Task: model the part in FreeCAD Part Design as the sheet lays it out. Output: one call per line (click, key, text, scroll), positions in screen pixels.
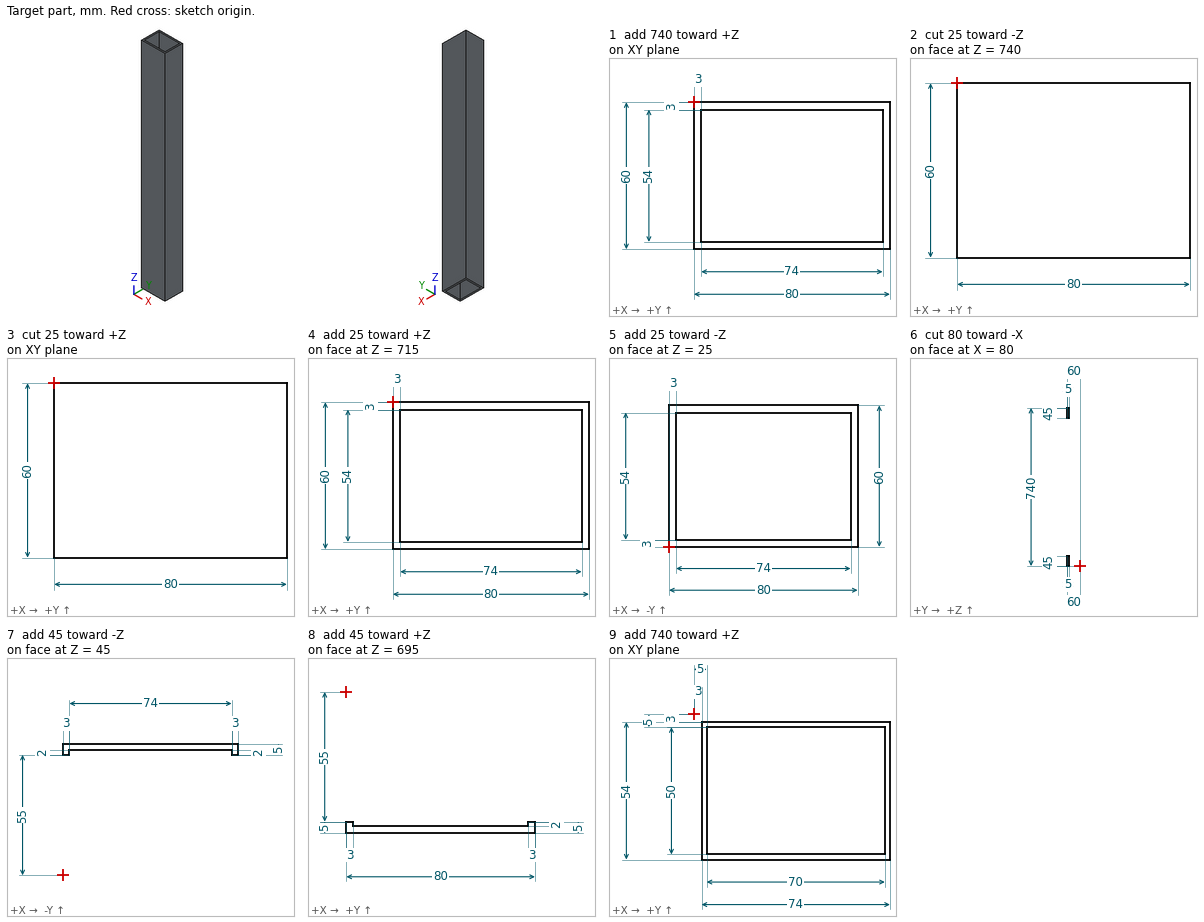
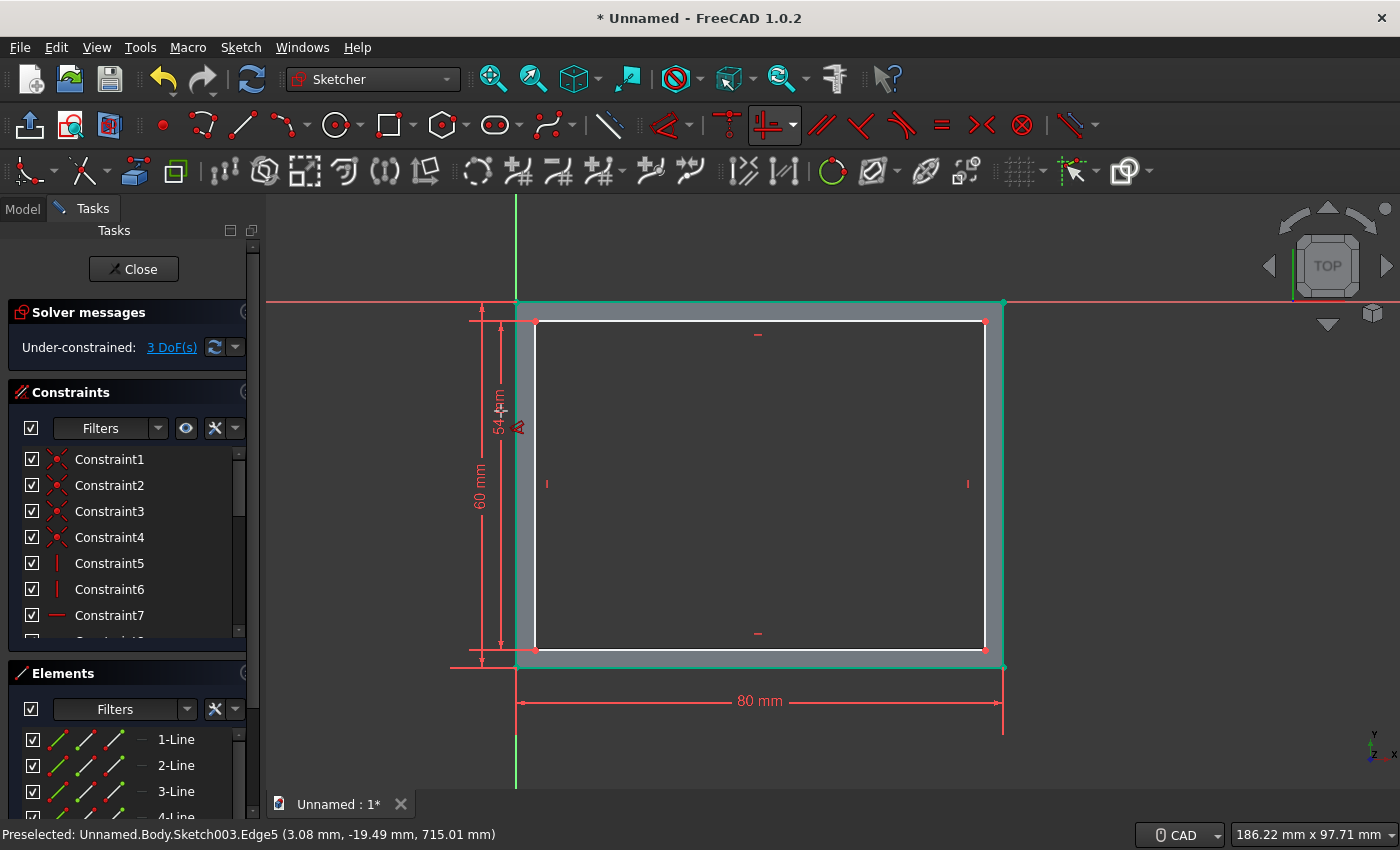
click(670, 650)
click(656, 684)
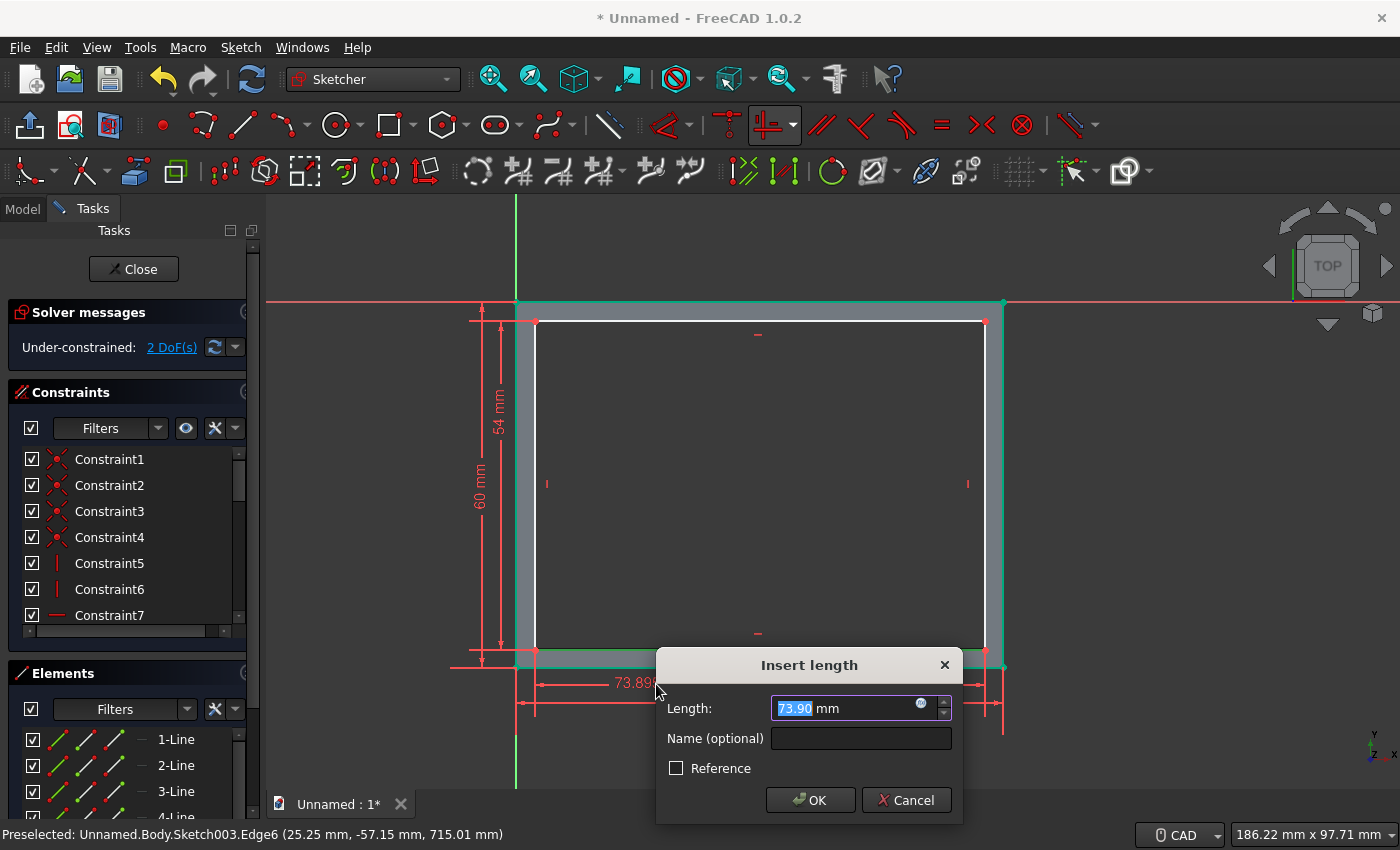
text(74)
key(Return)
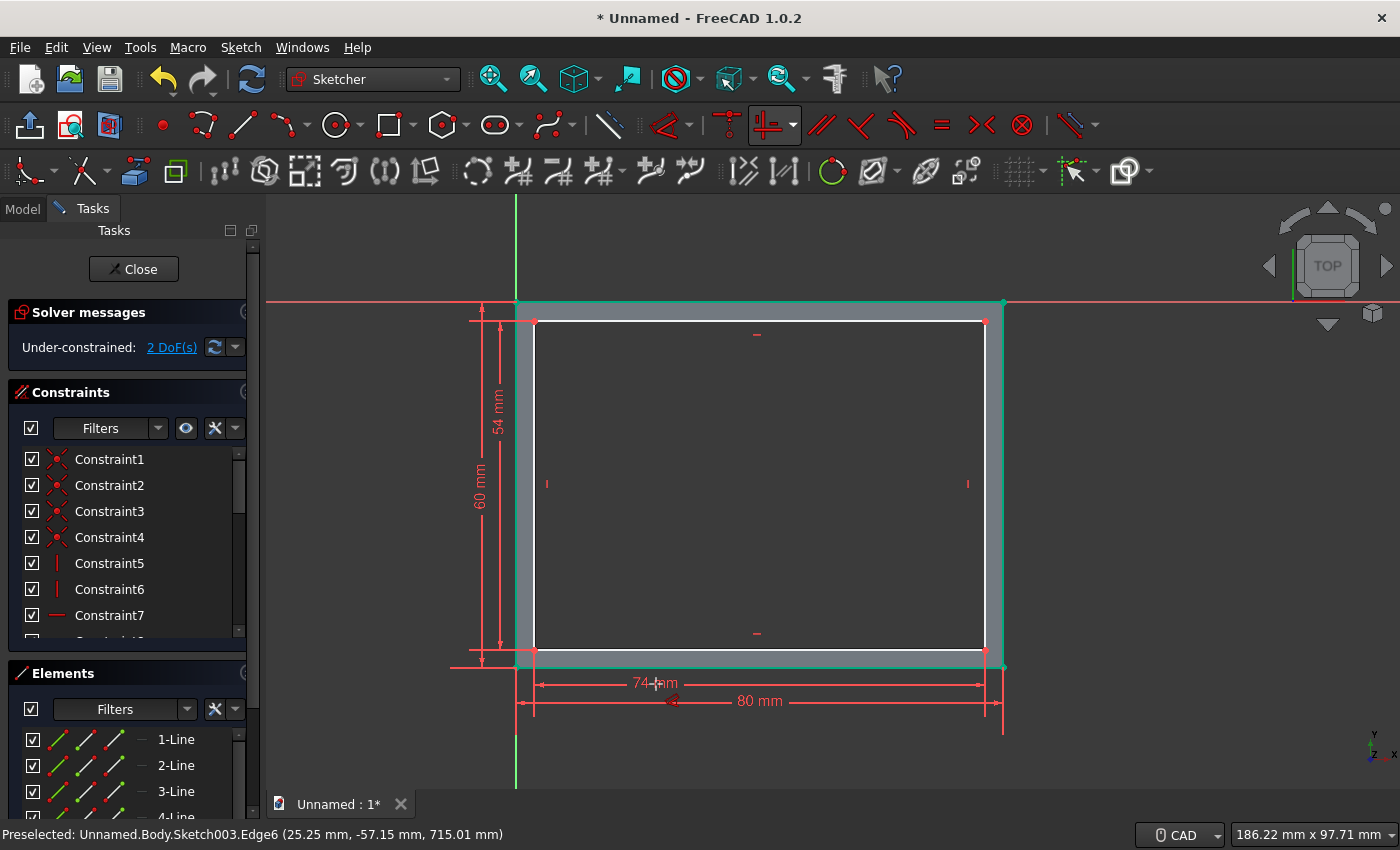
scroll(534, 321, up, 4)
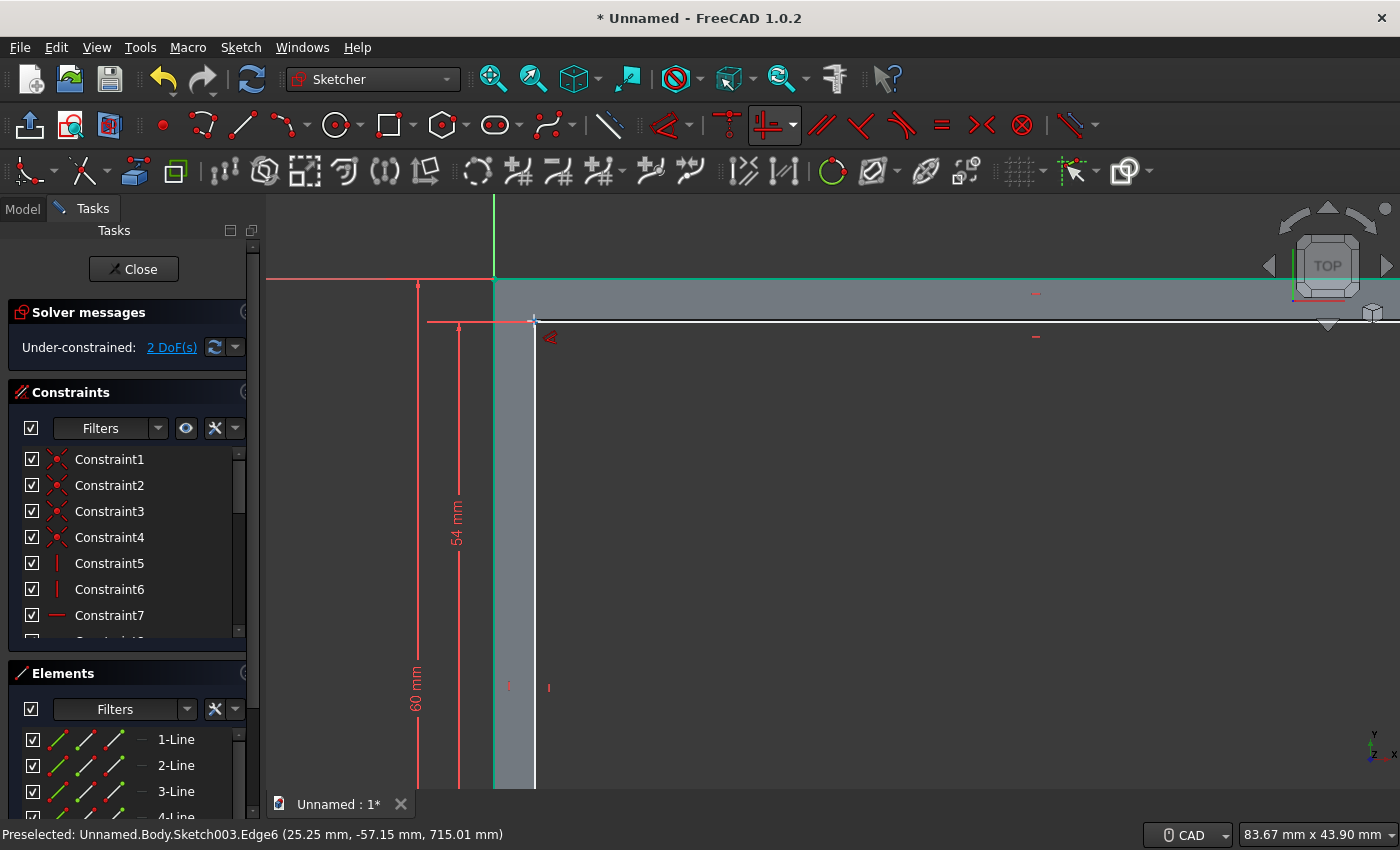
click(535, 322)
click(514, 245)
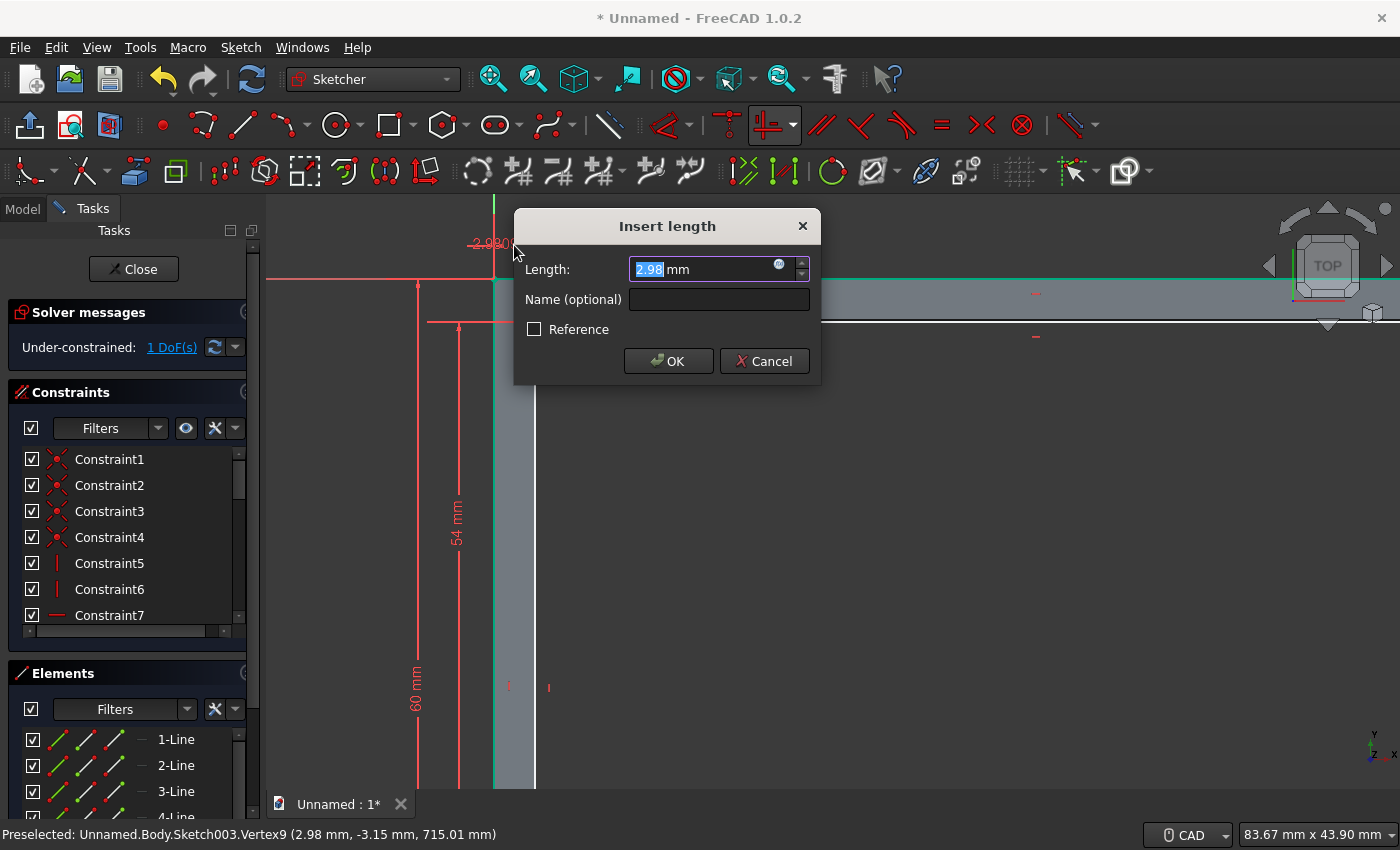
text(3)
key(Return)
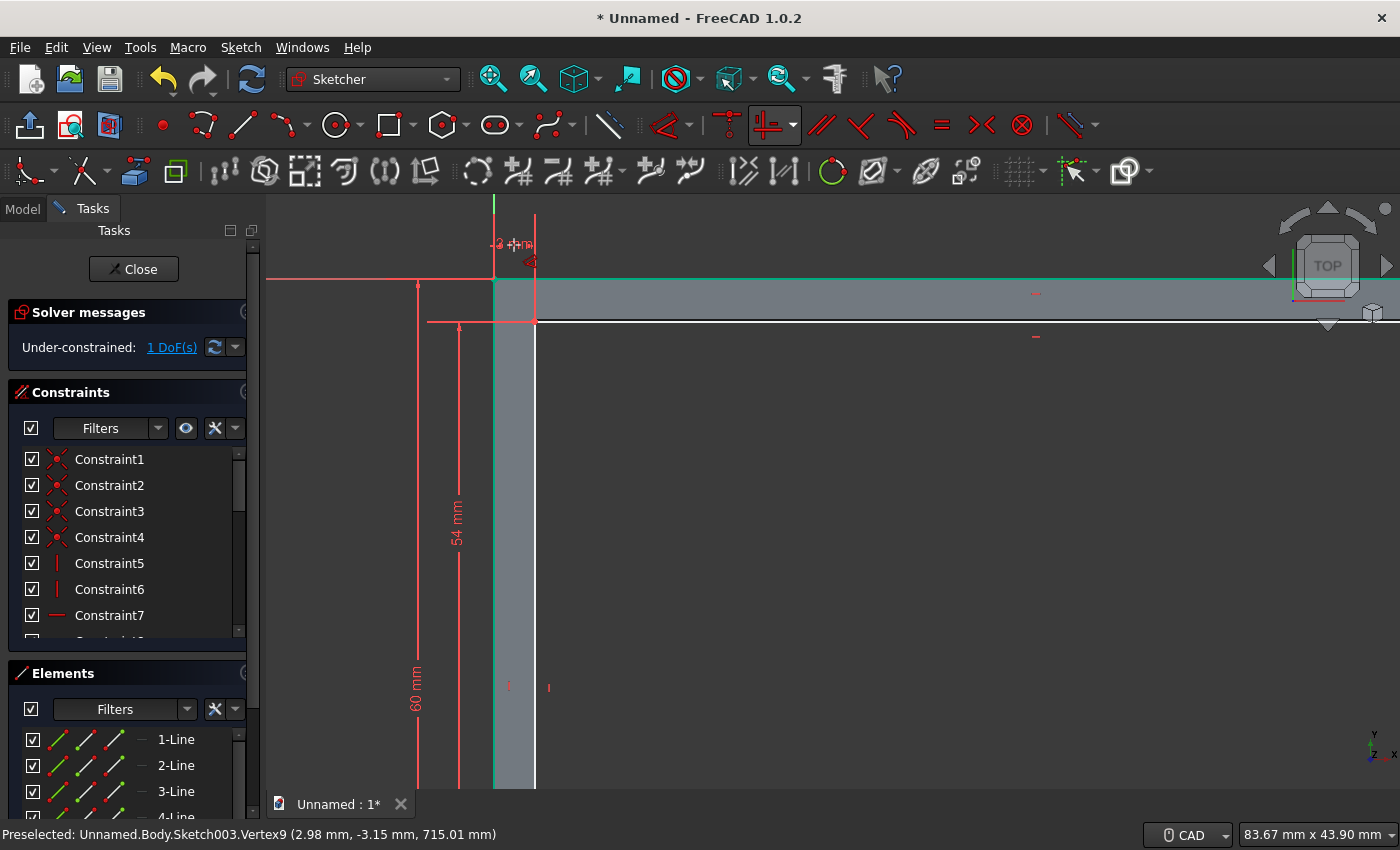
click(535, 322)
click(460, 300)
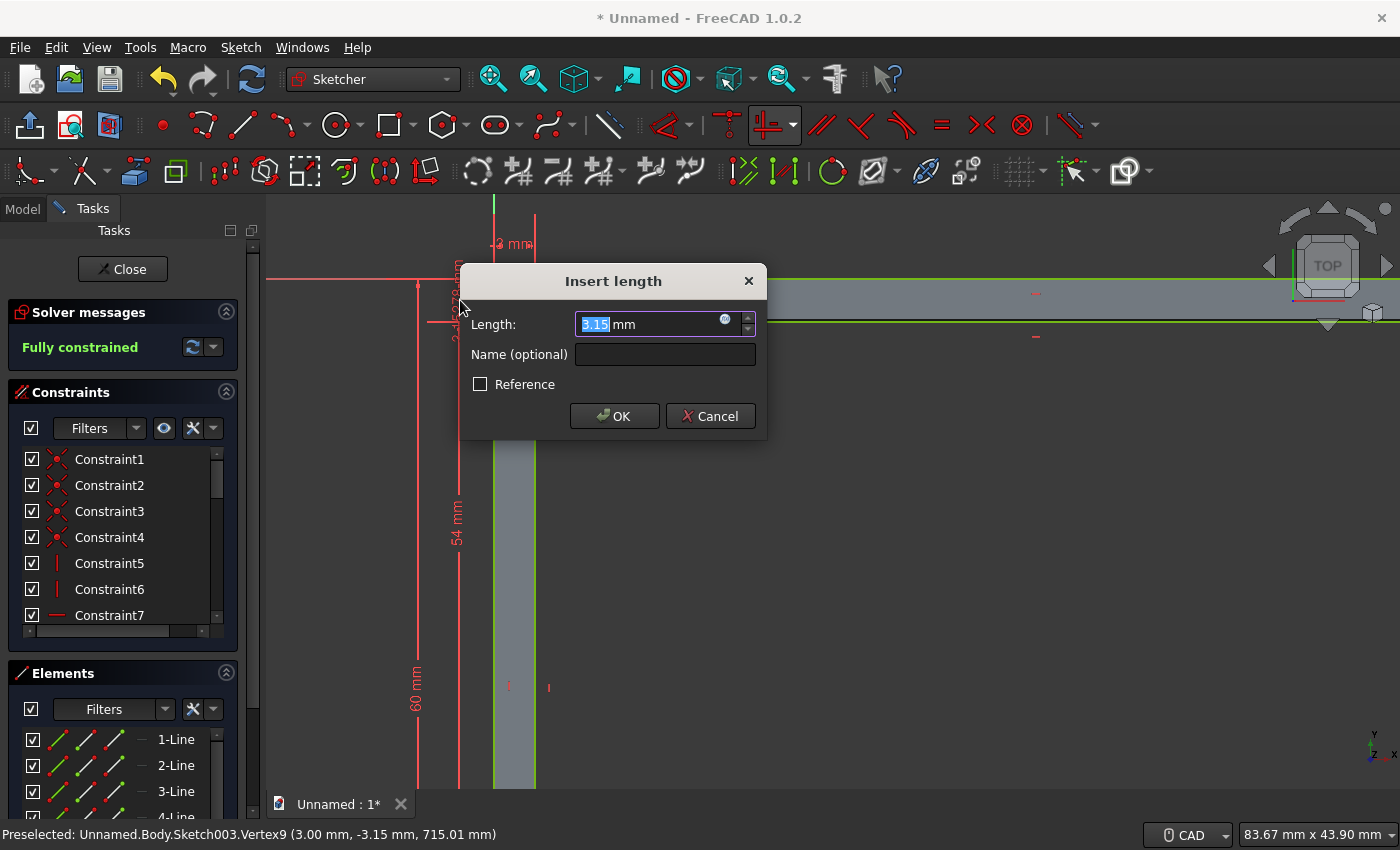
text(3)
key(Return)
key(Escape)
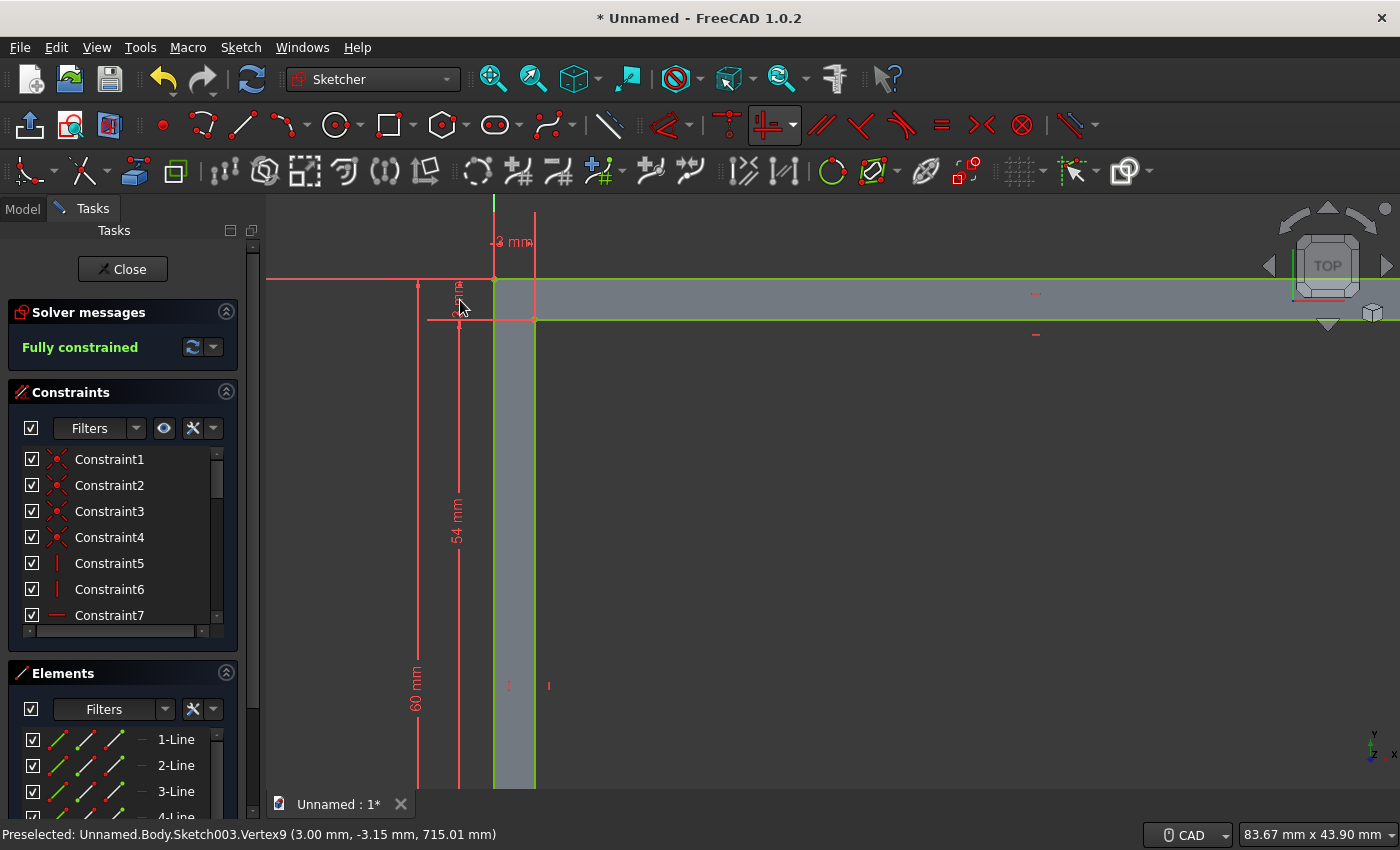
click(123, 269)